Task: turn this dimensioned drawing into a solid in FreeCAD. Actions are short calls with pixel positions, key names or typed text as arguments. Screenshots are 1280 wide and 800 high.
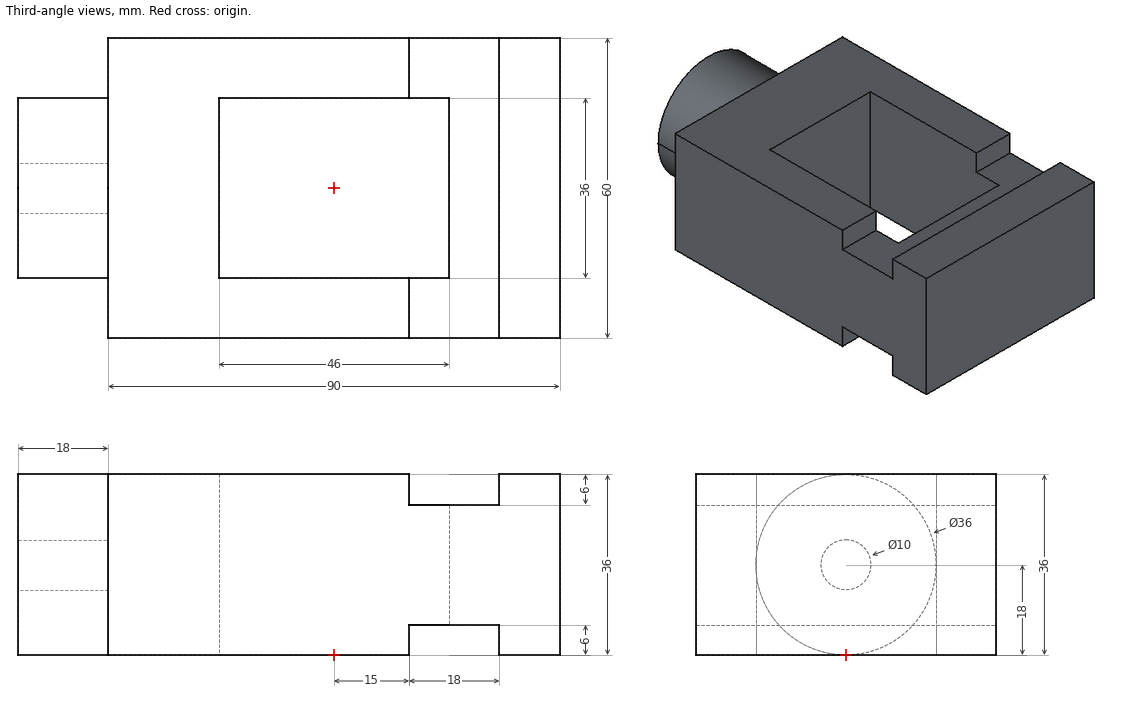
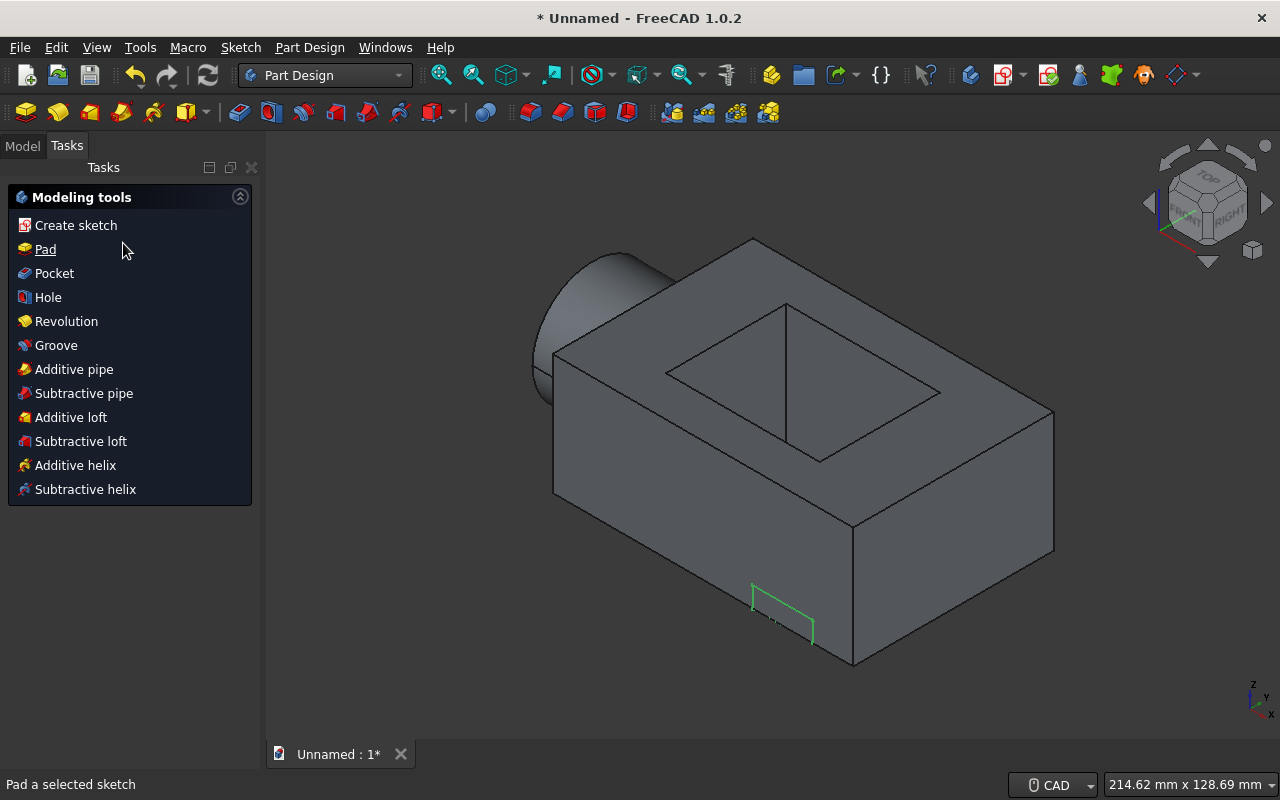
click(240, 112)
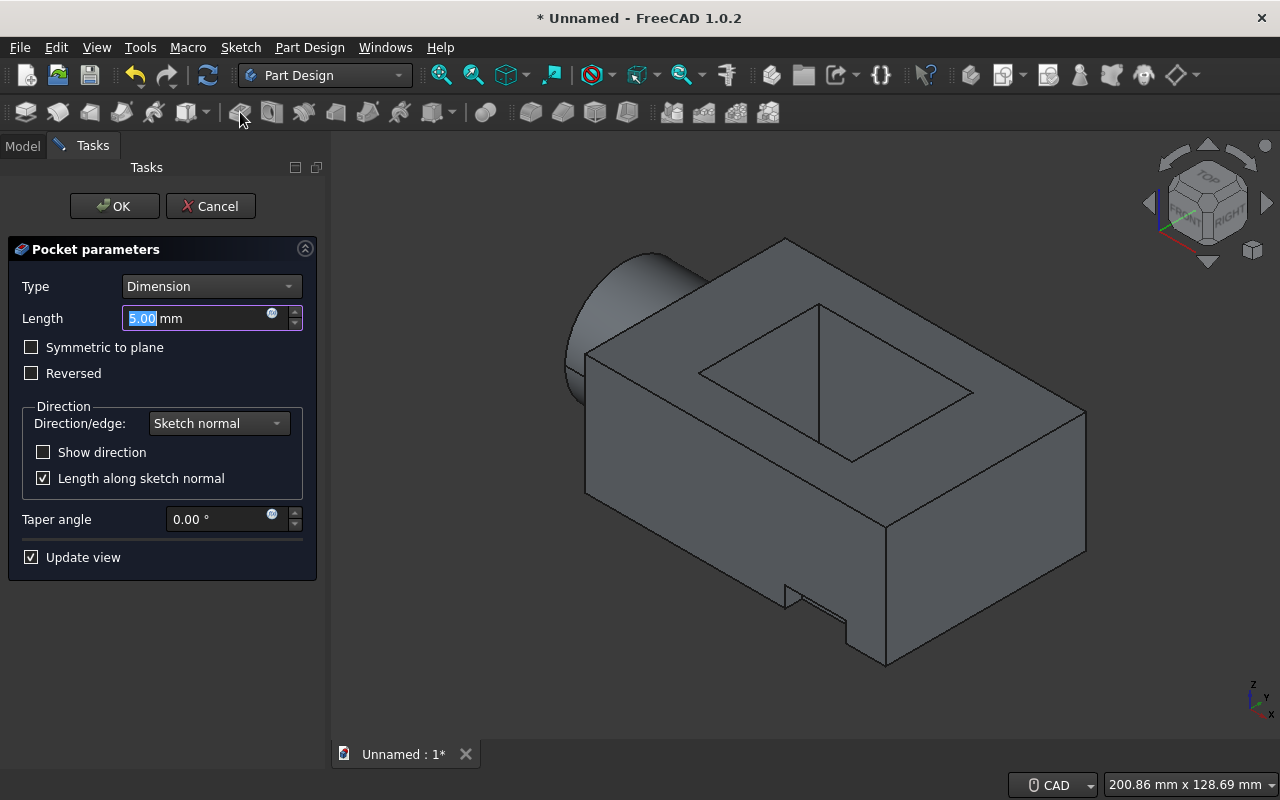
click(212, 286)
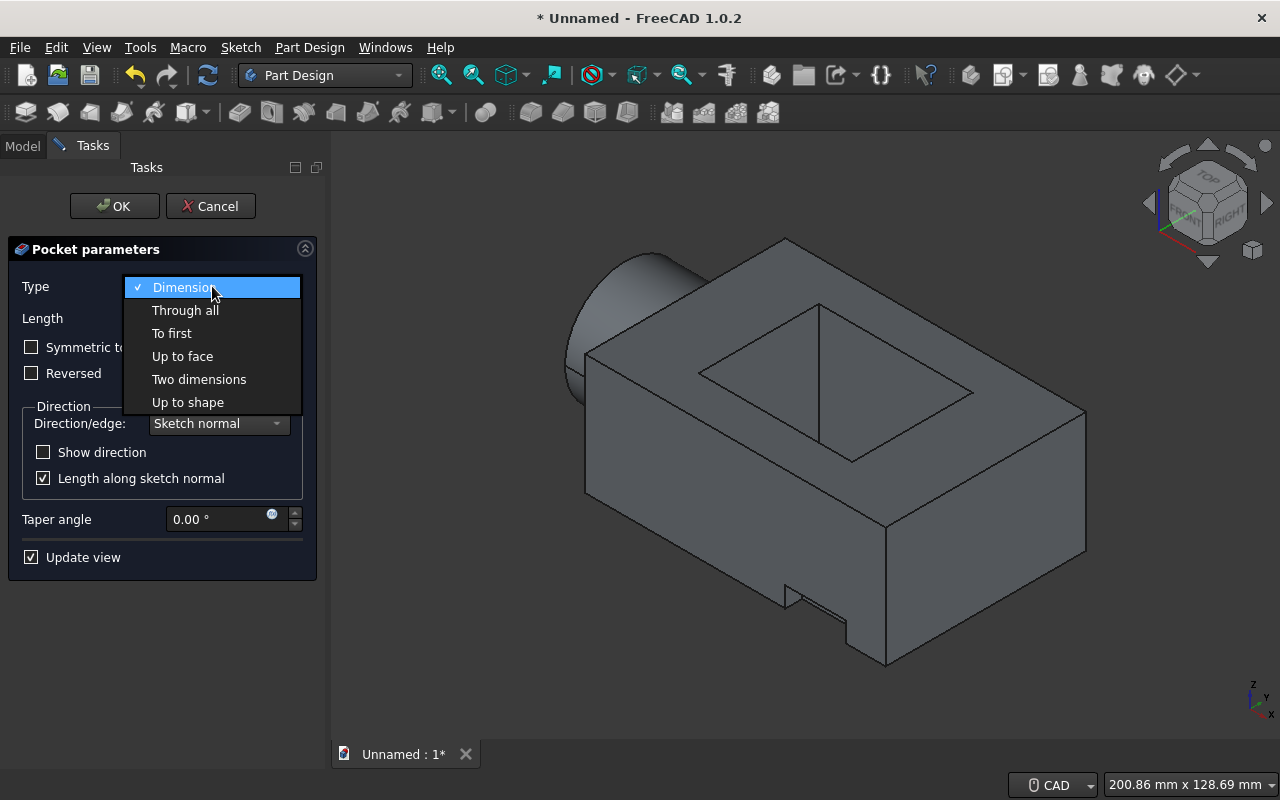
click(212, 310)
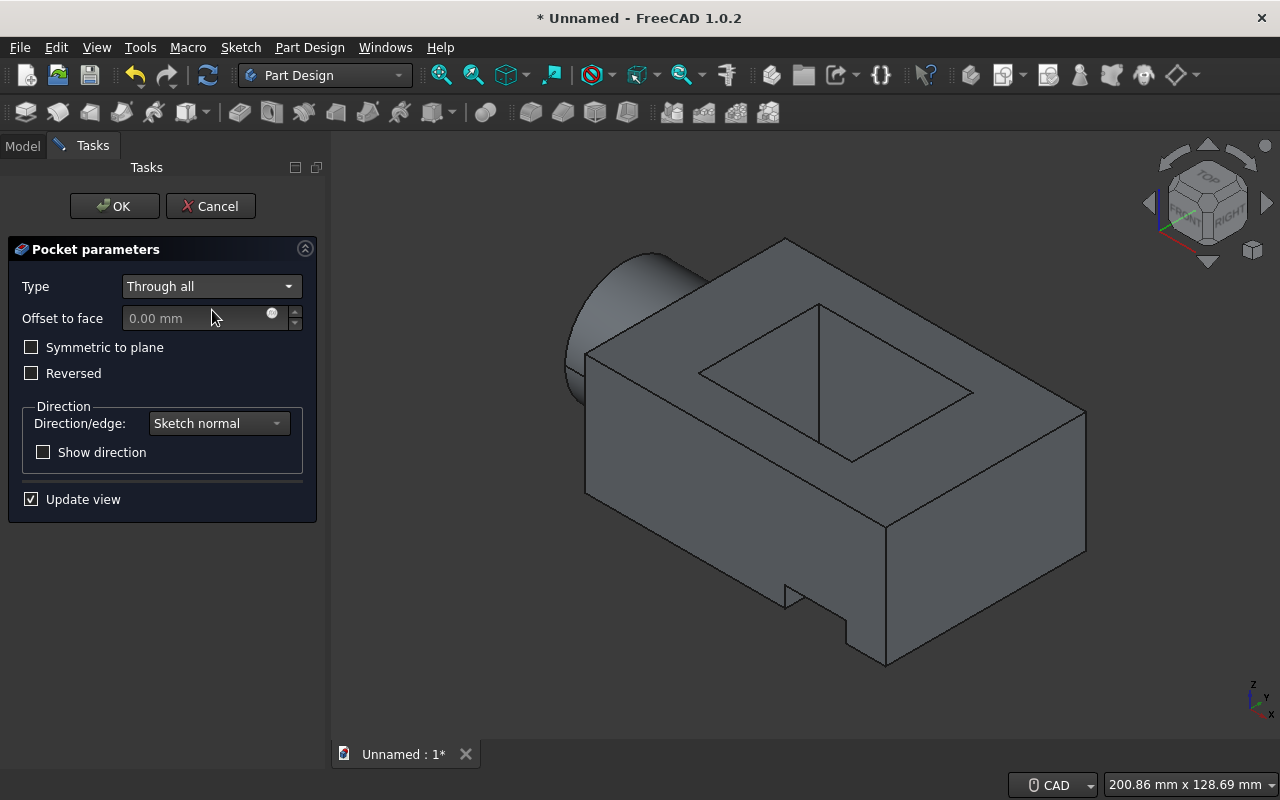
click(115, 206)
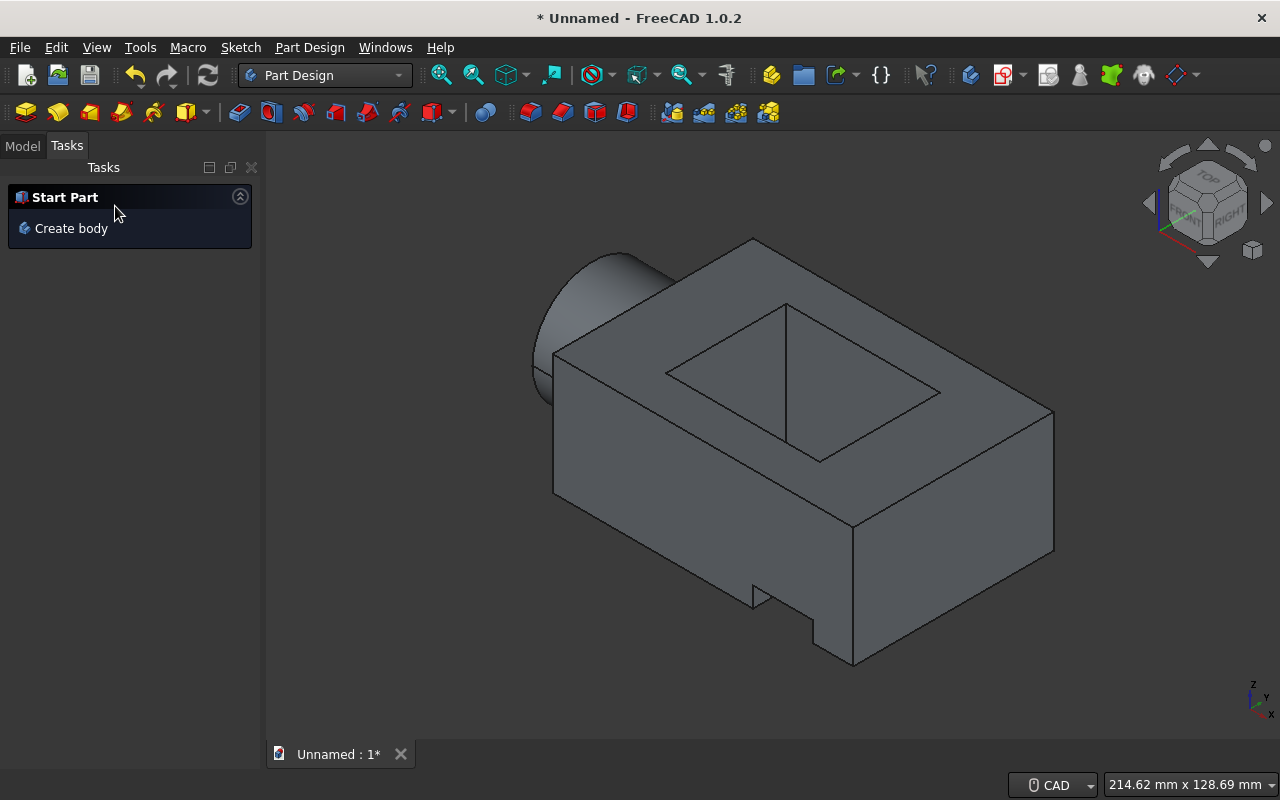
click(703, 509)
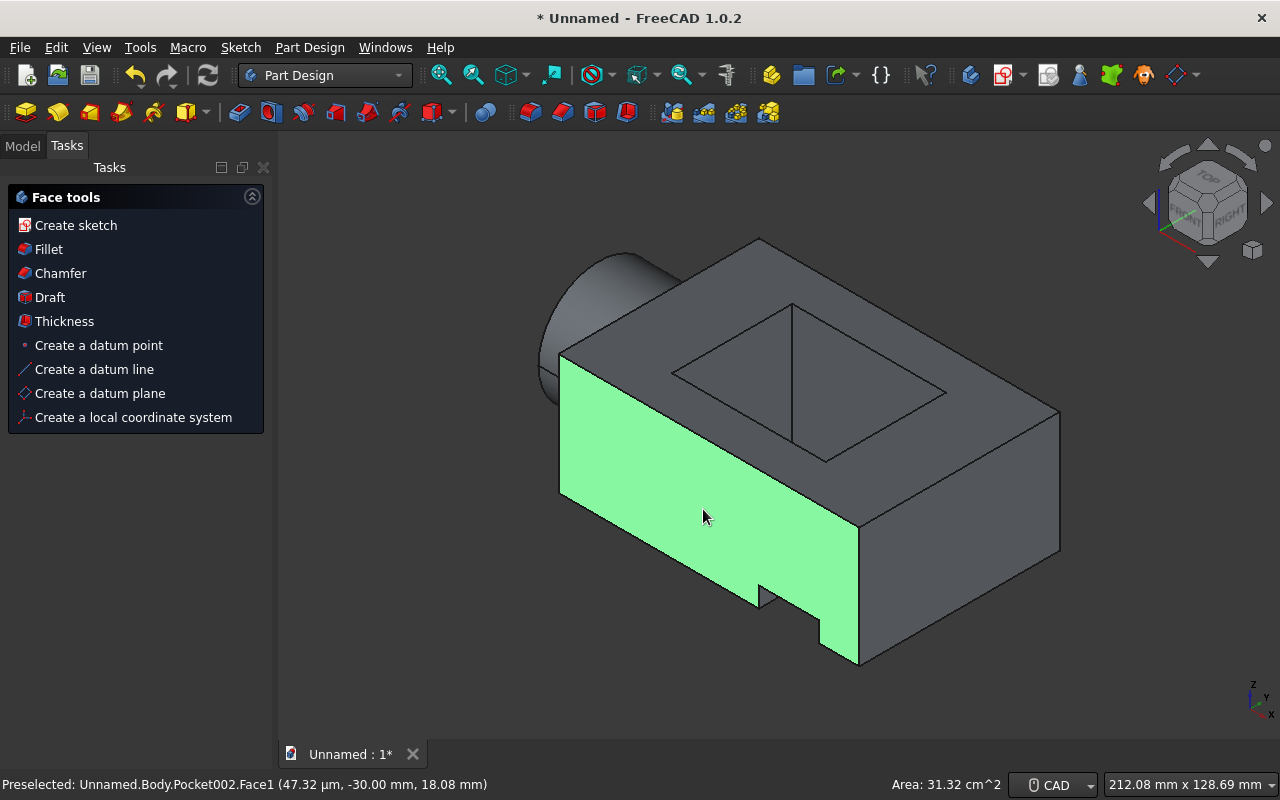
click(1004, 76)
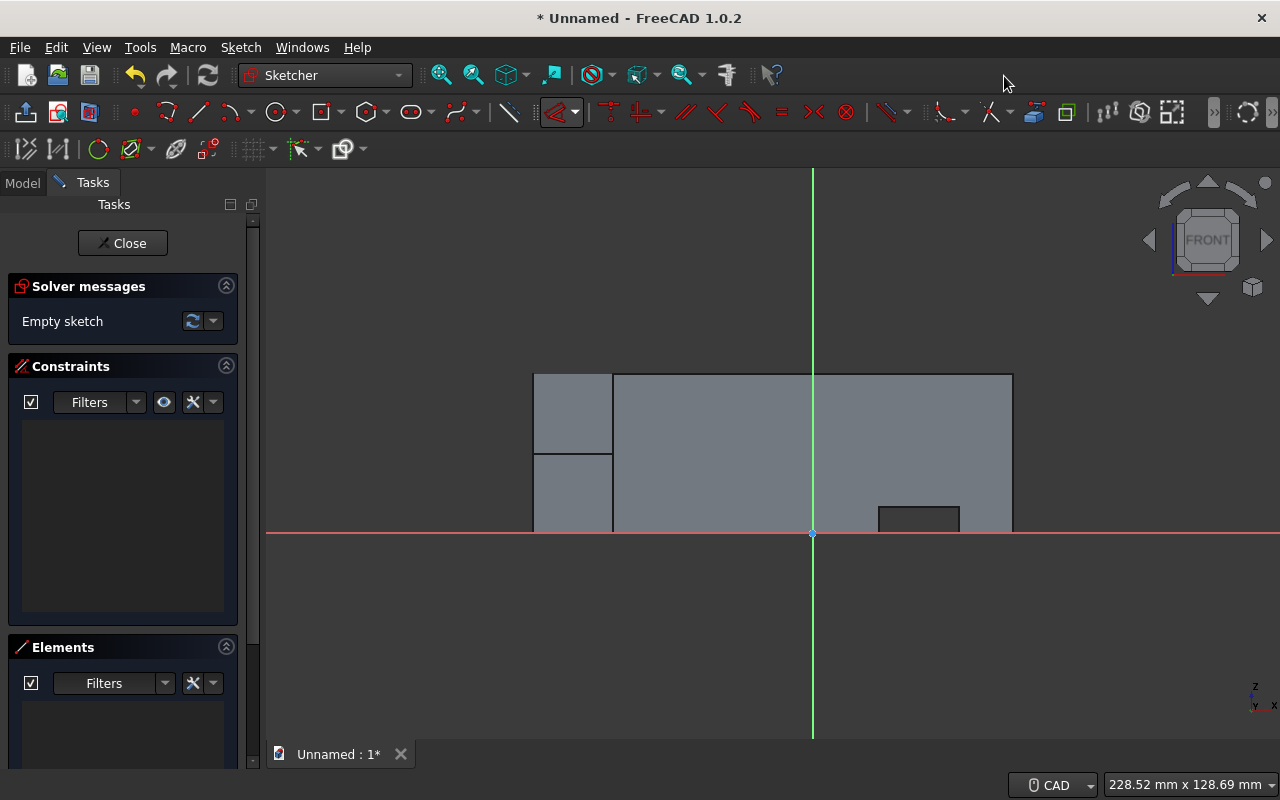
scroll(1034, 453, up, 4)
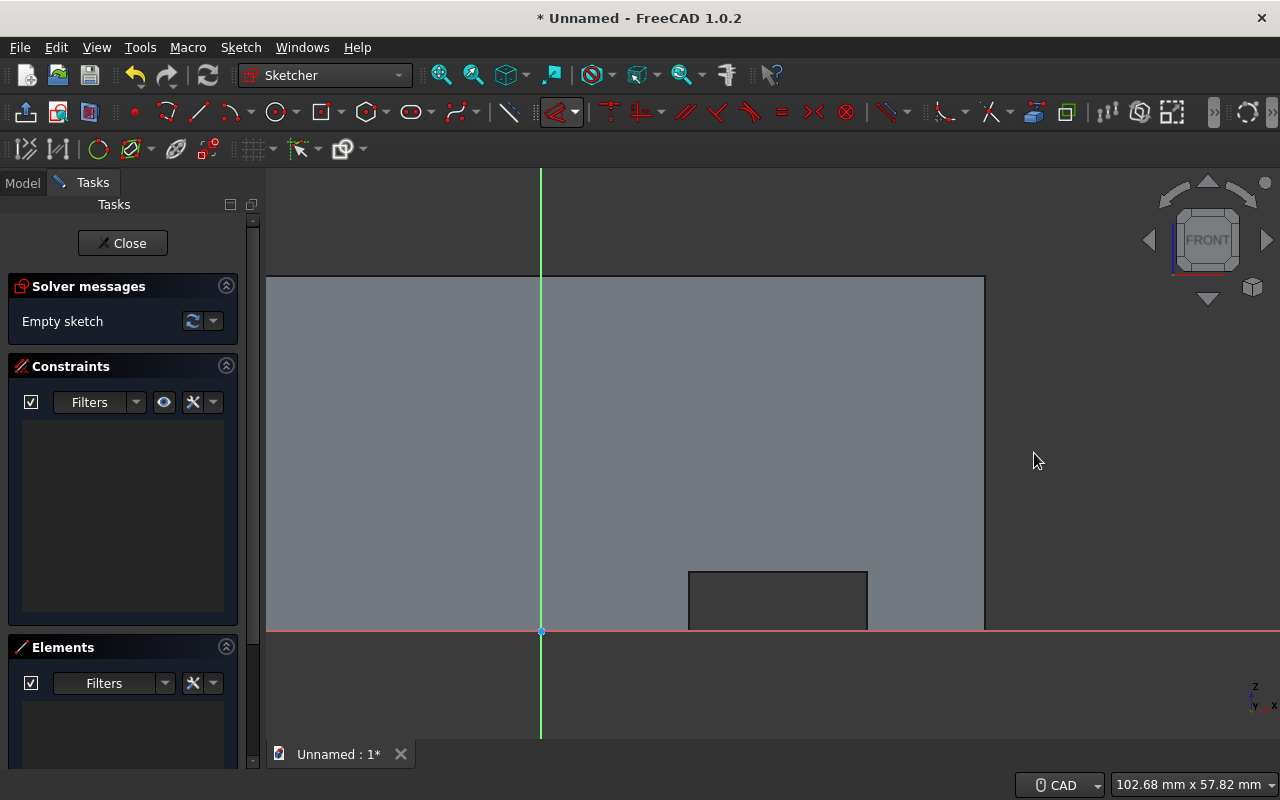
key(g)
key(r)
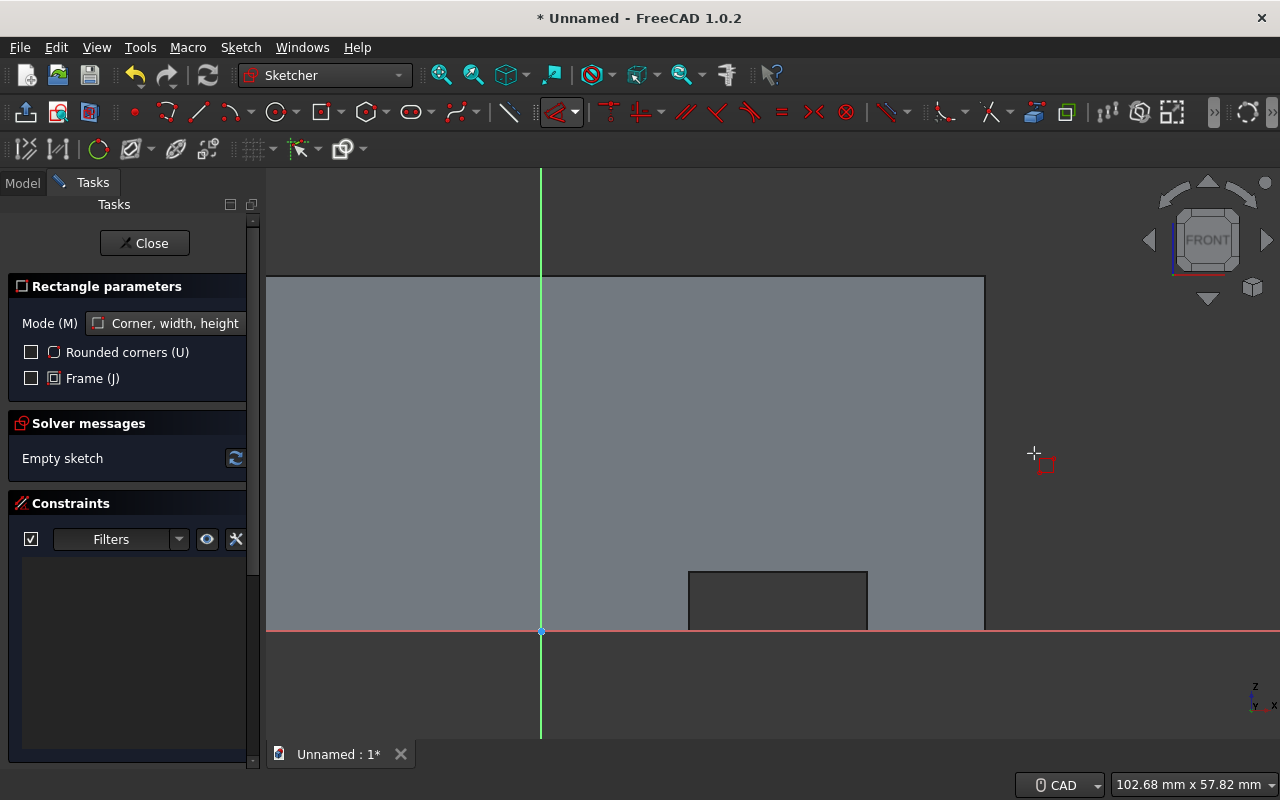
click(689, 276)
click(867, 335)
key(Escape)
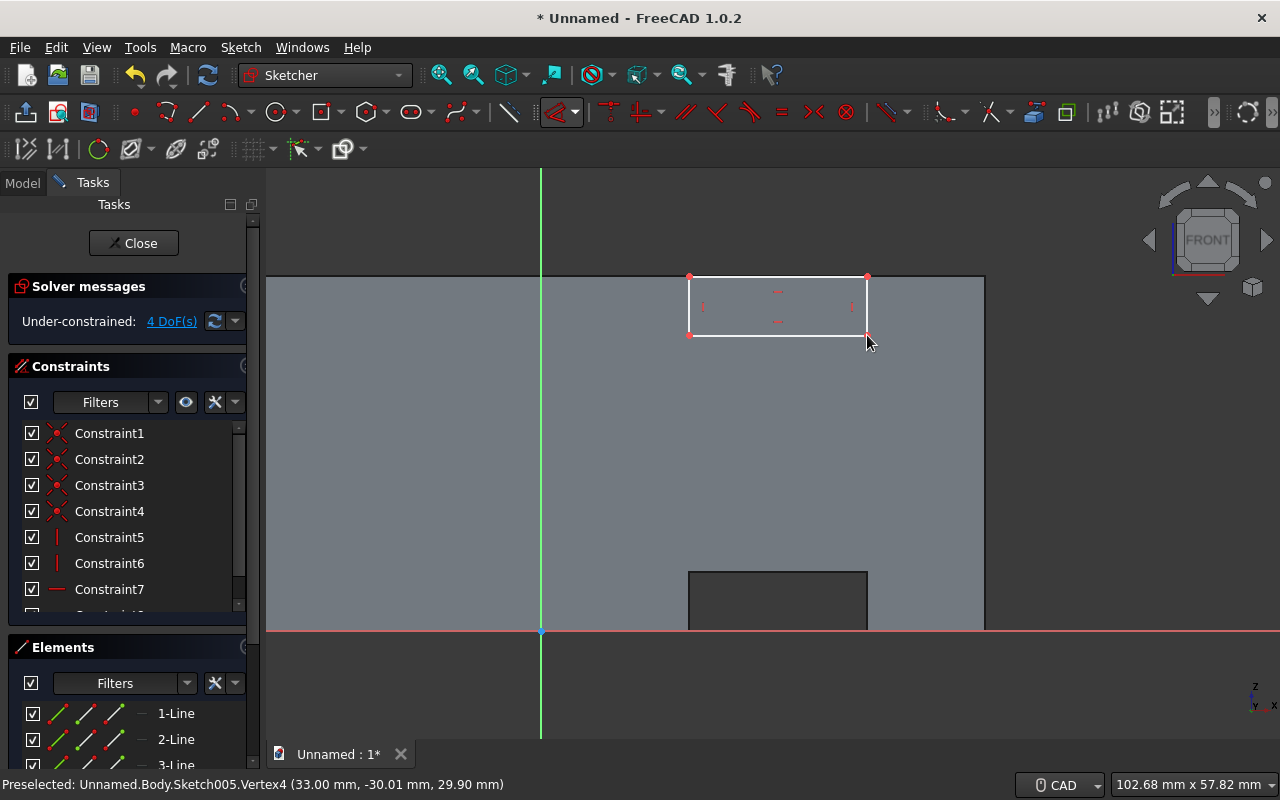
click(689, 295)